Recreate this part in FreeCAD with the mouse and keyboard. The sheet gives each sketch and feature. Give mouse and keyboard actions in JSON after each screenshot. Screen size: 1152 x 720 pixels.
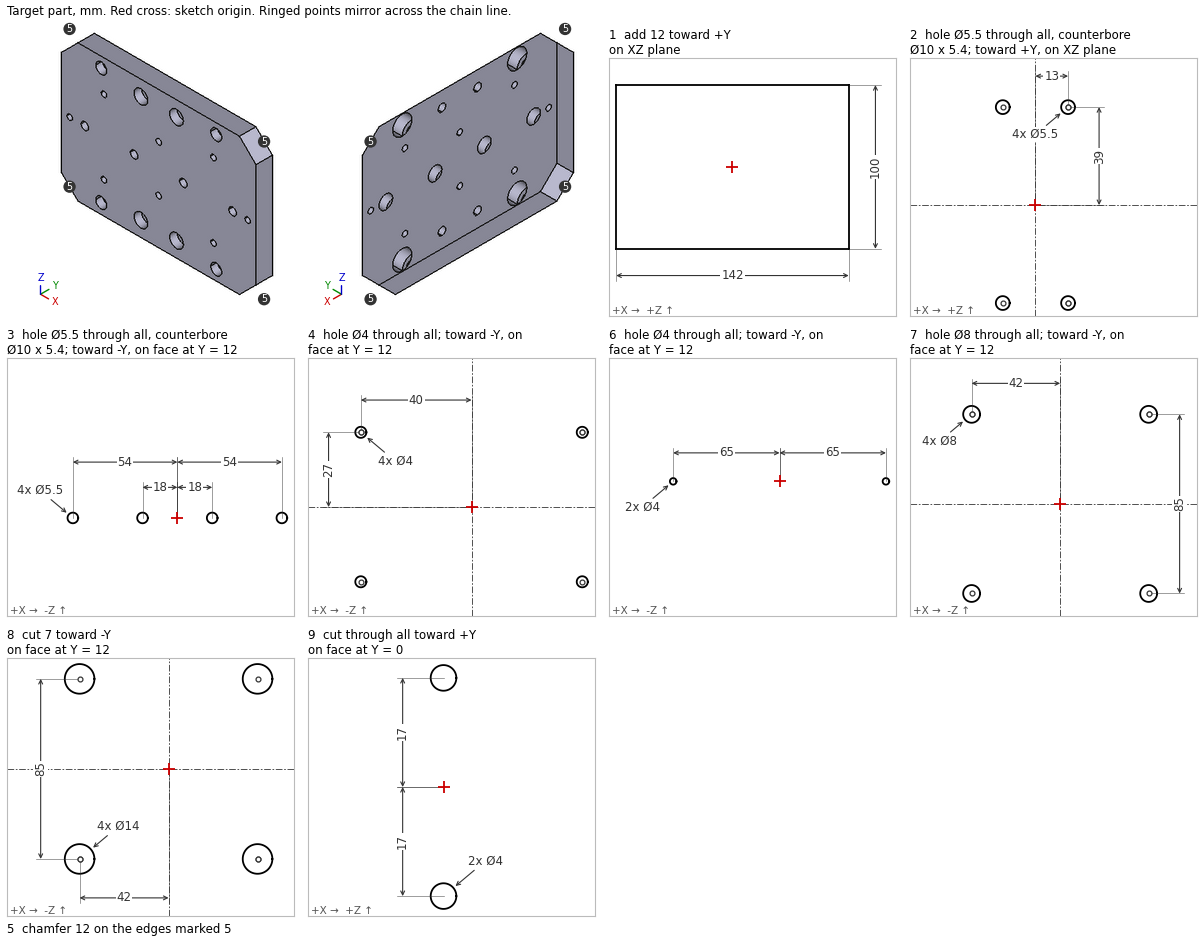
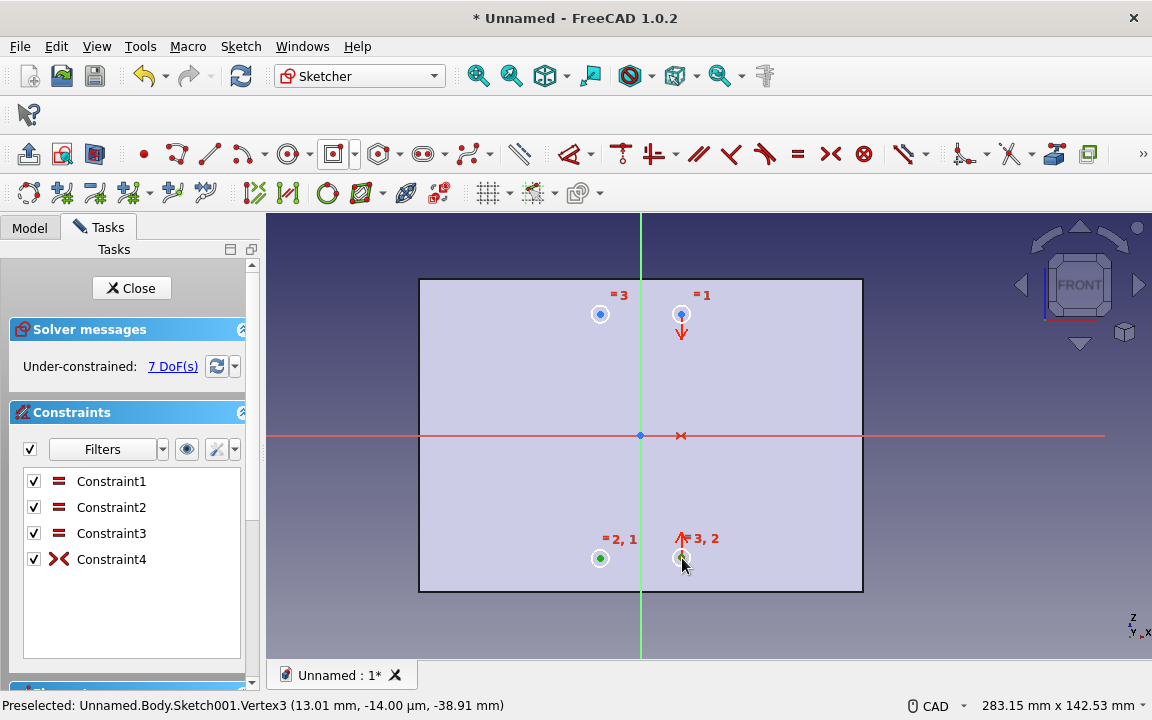
{"action": "left_click", "coordinate": [641, 603]}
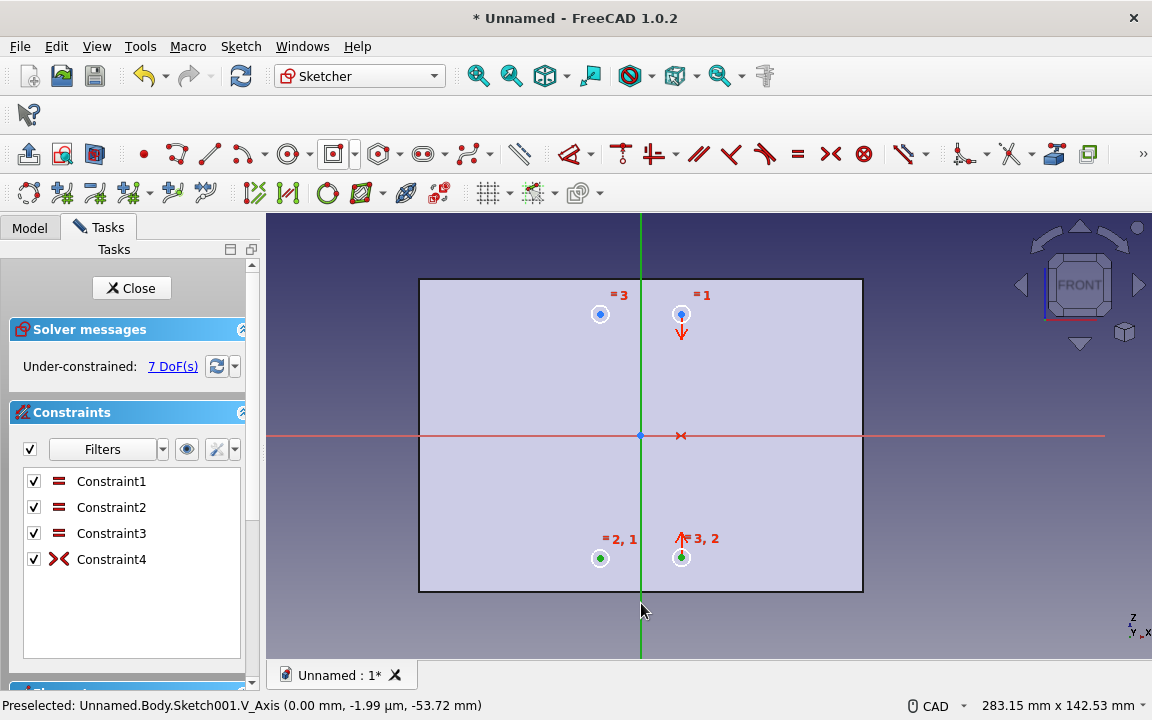
{"action": "left_click", "coordinate": [831, 154]}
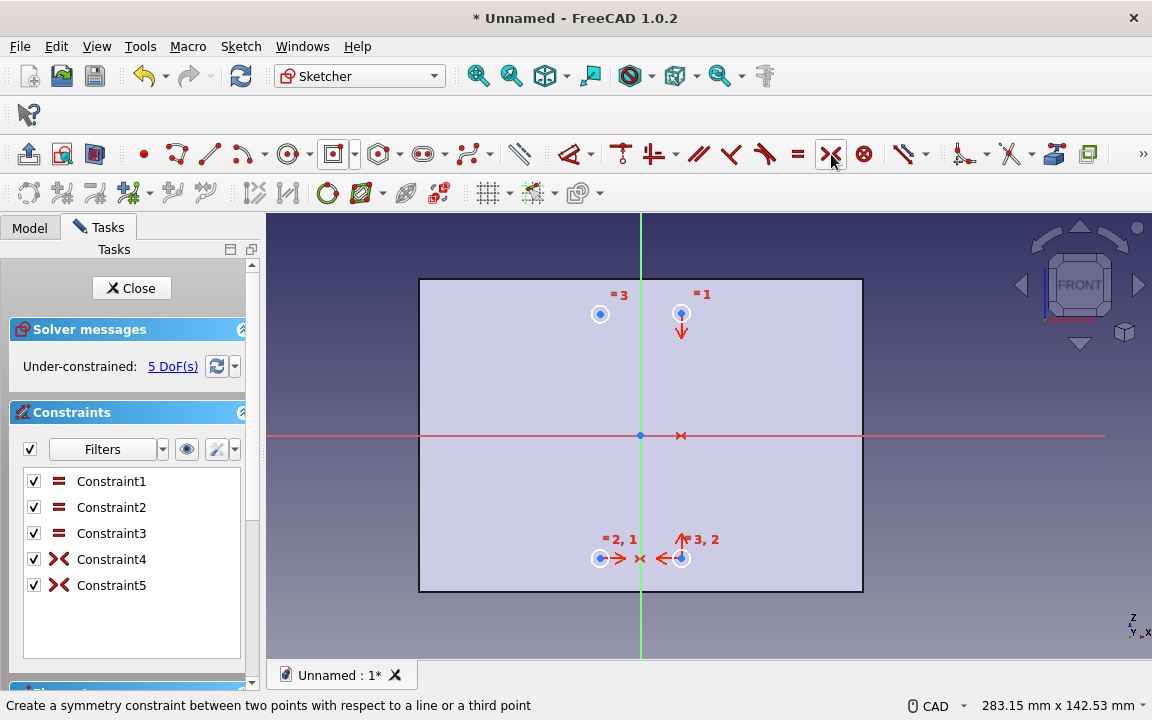
{"action": "left_click", "coordinate": [682, 313]}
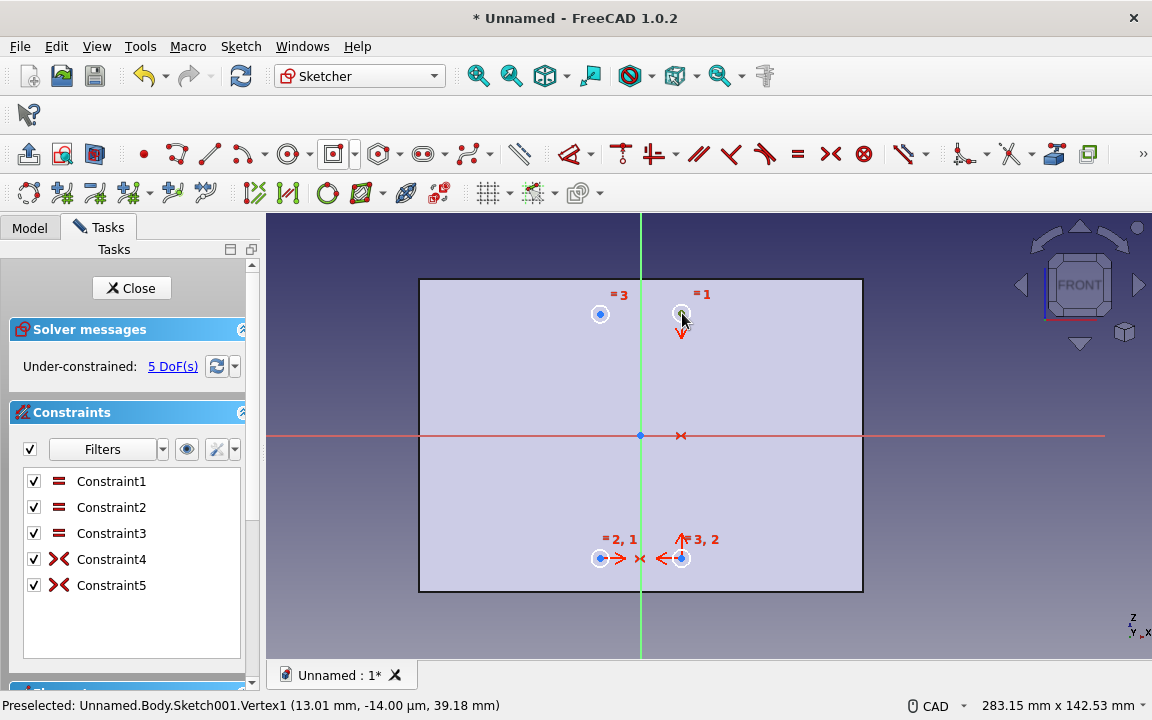
{"action": "left_click", "coordinate": [600, 314]}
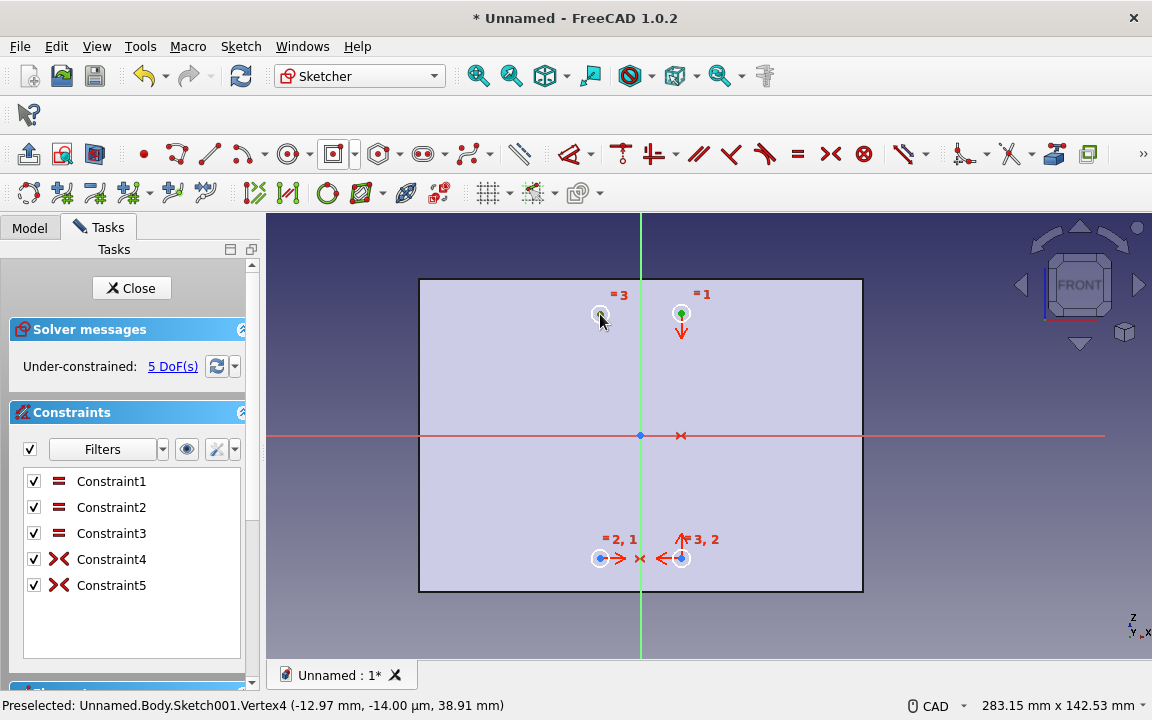
{"action": "left_click", "coordinate": [641, 603]}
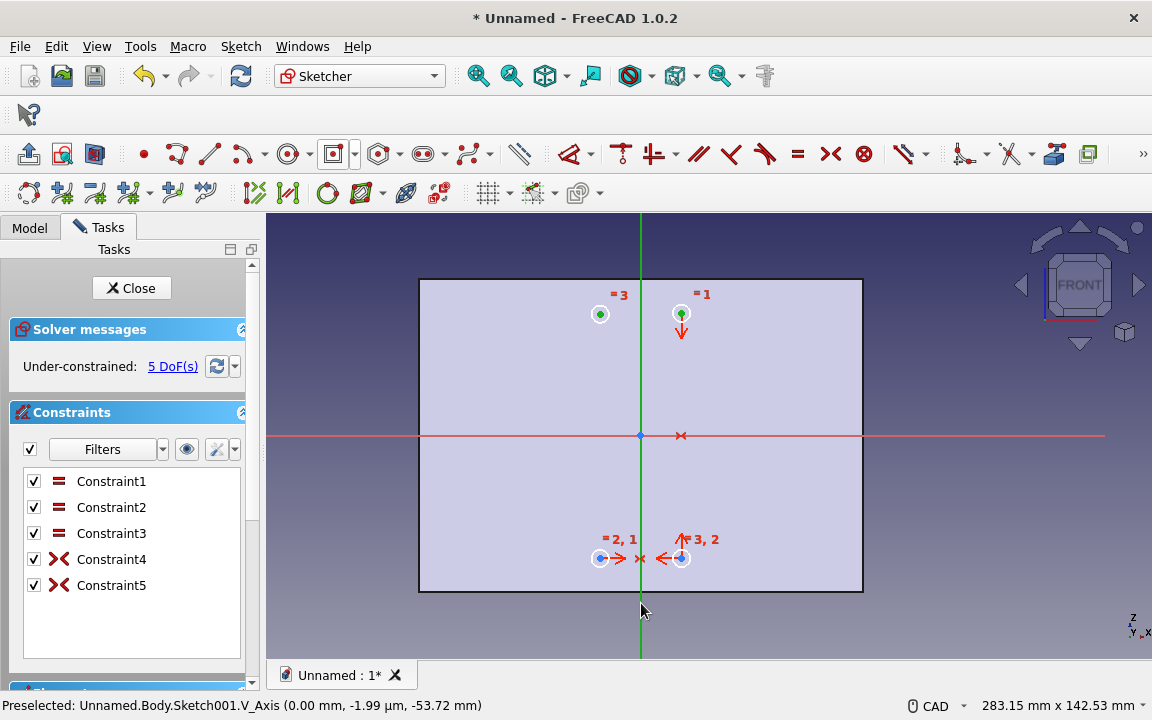
{"action": "left_click", "coordinate": [831, 154]}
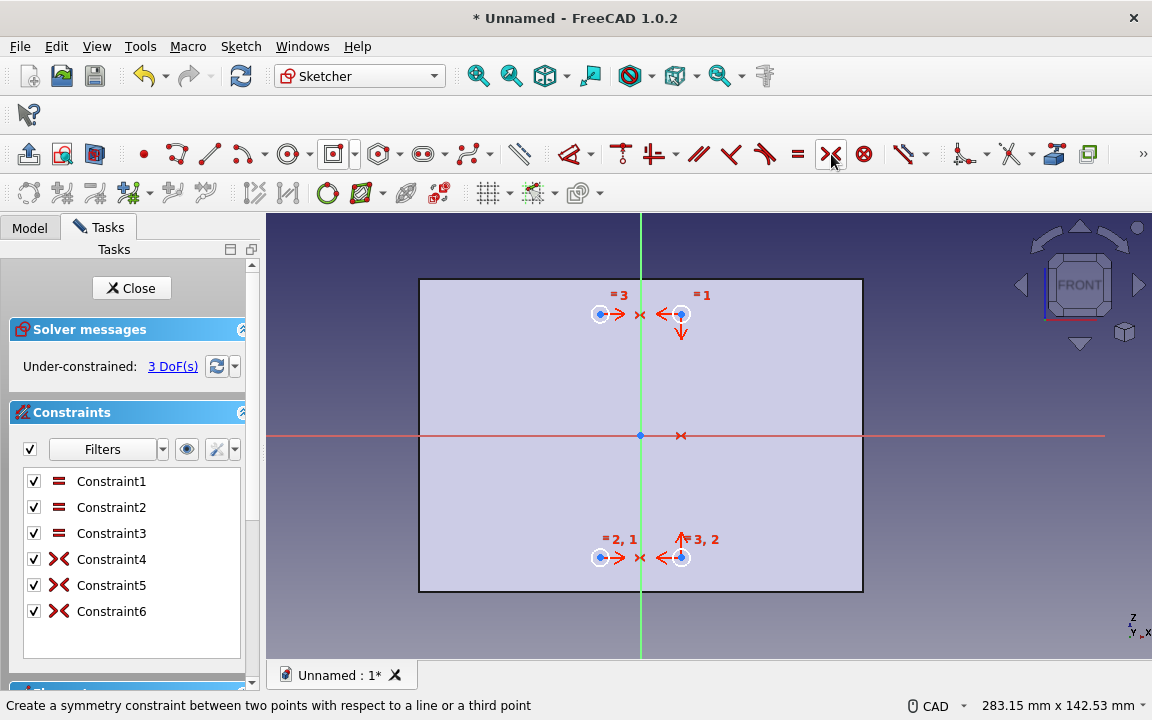
{"action": "left_click", "coordinate": [568, 154]}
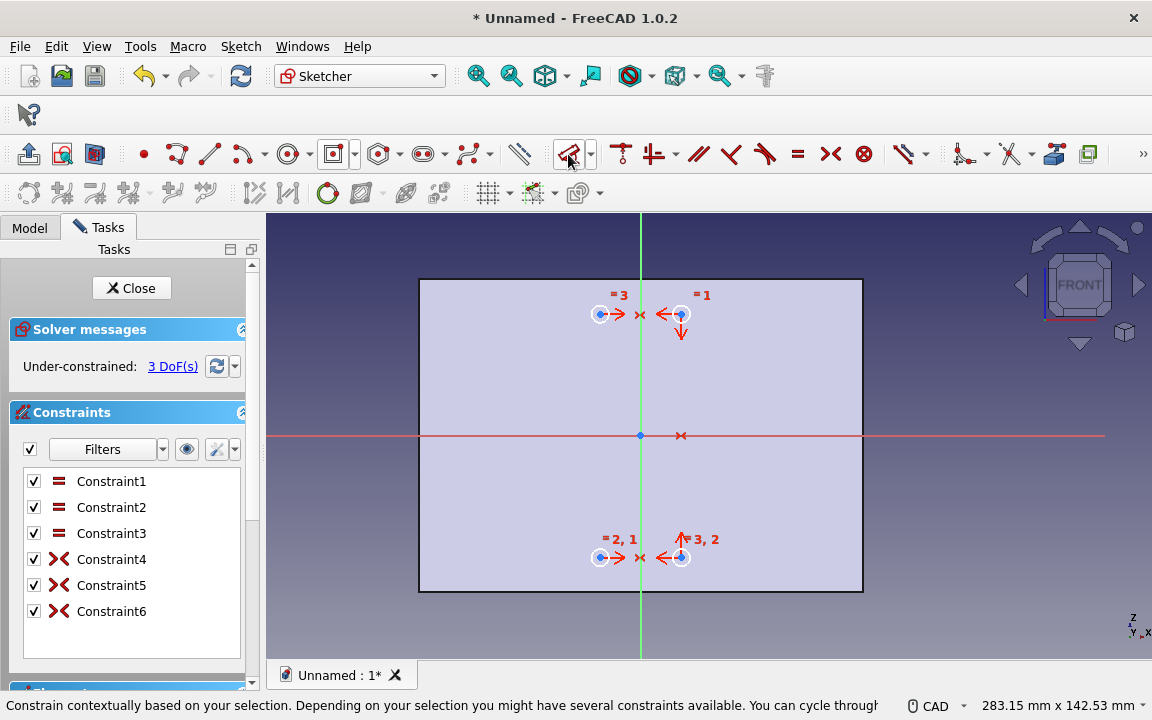
{"action": "scroll", "coordinate": [675, 308], "scroll_direction": "up", "scroll_amount": 5}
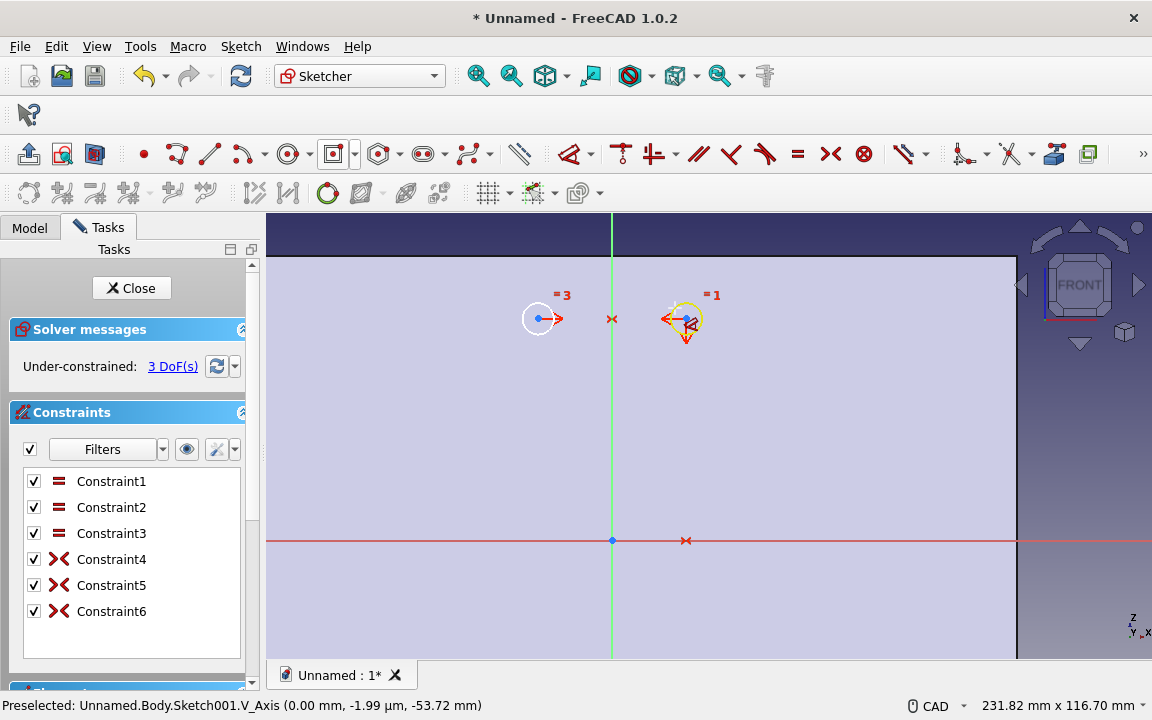
{"action": "left_click", "coordinate": [675, 308]}
{"action": "left_click", "coordinate": [652, 286]}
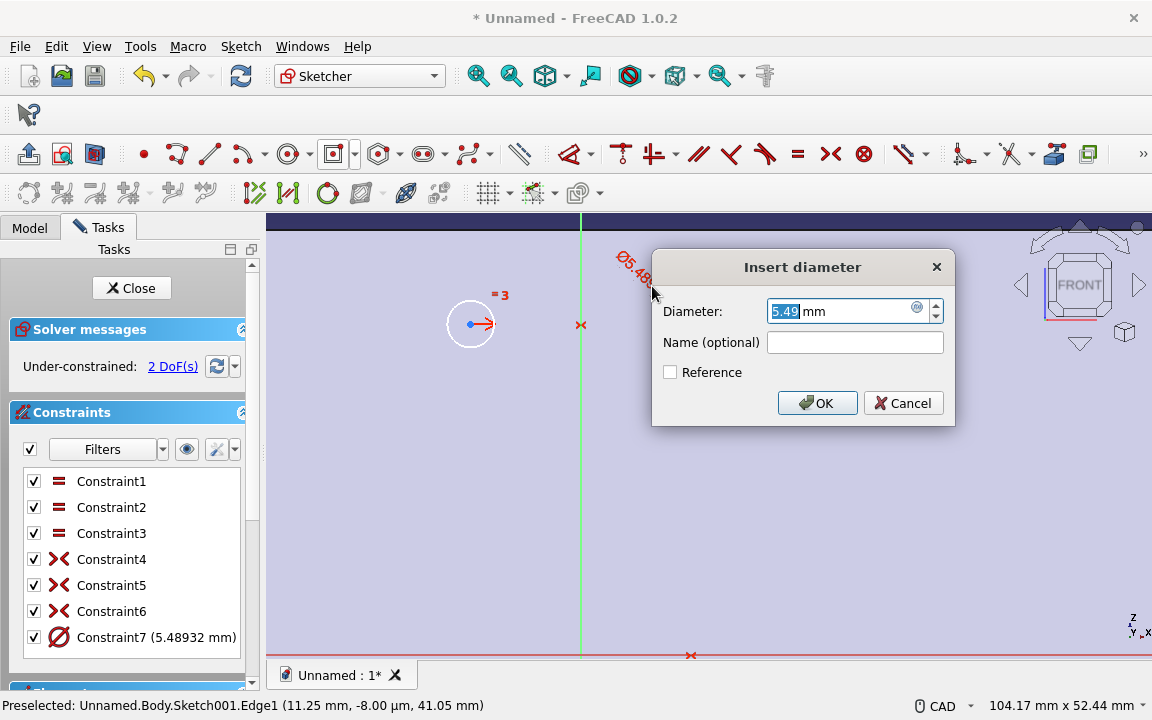
{"action": "type", "text": "5.5"}
{"action": "key", "text": "Return"}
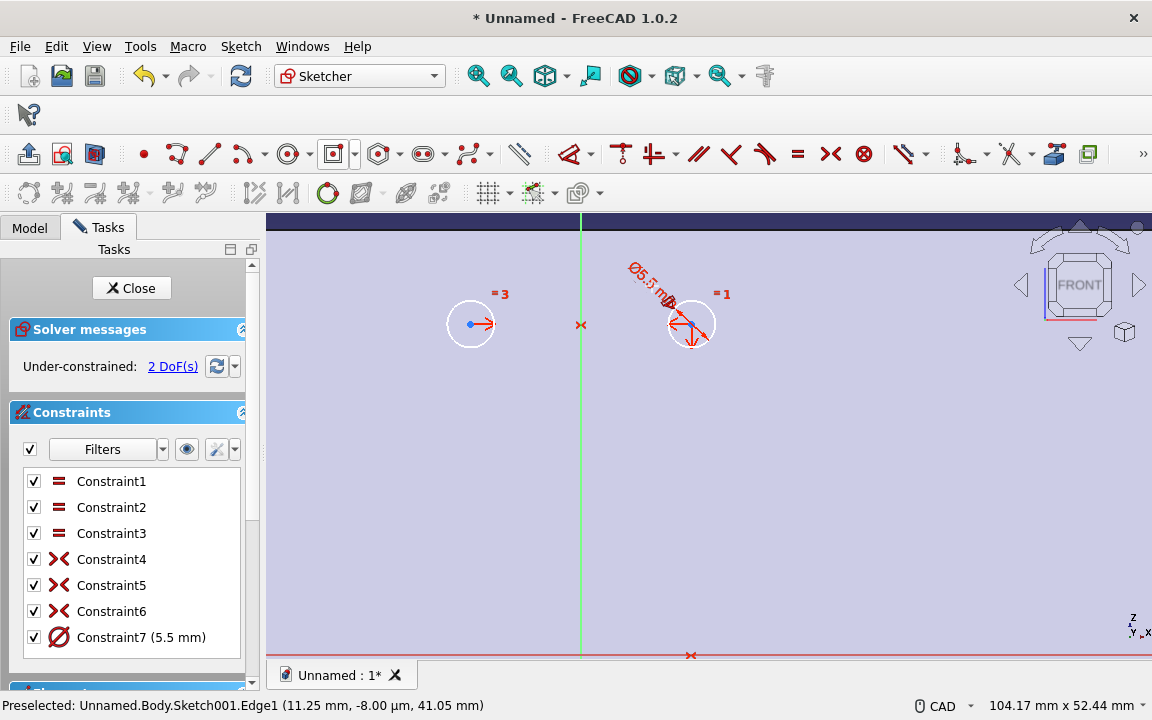
{"action": "left_click", "coordinate": [692, 324]}
{"action": "left_click", "coordinate": [637, 242]}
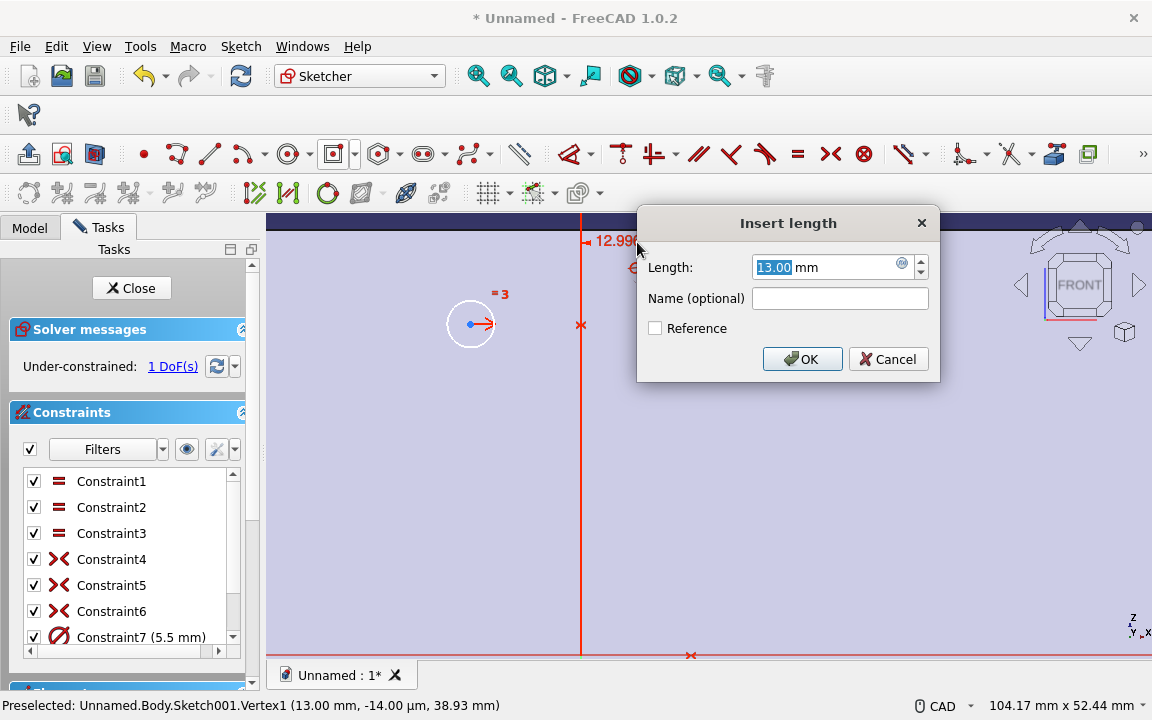
{"action": "type", "text": "13"}
{"action": "key", "text": "Return"}